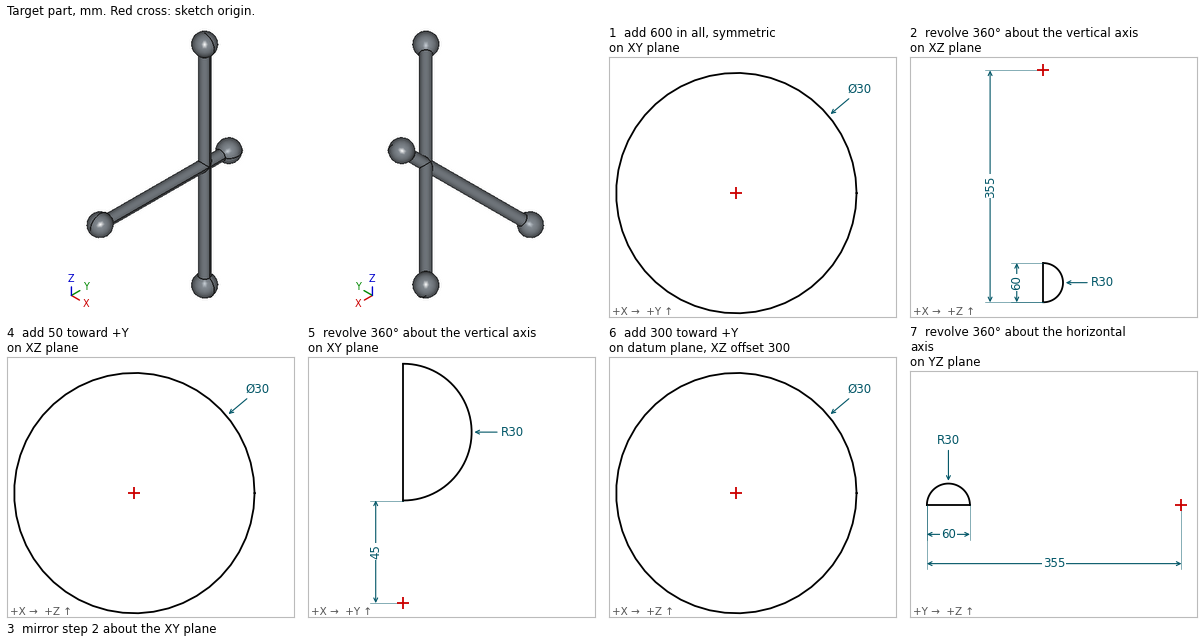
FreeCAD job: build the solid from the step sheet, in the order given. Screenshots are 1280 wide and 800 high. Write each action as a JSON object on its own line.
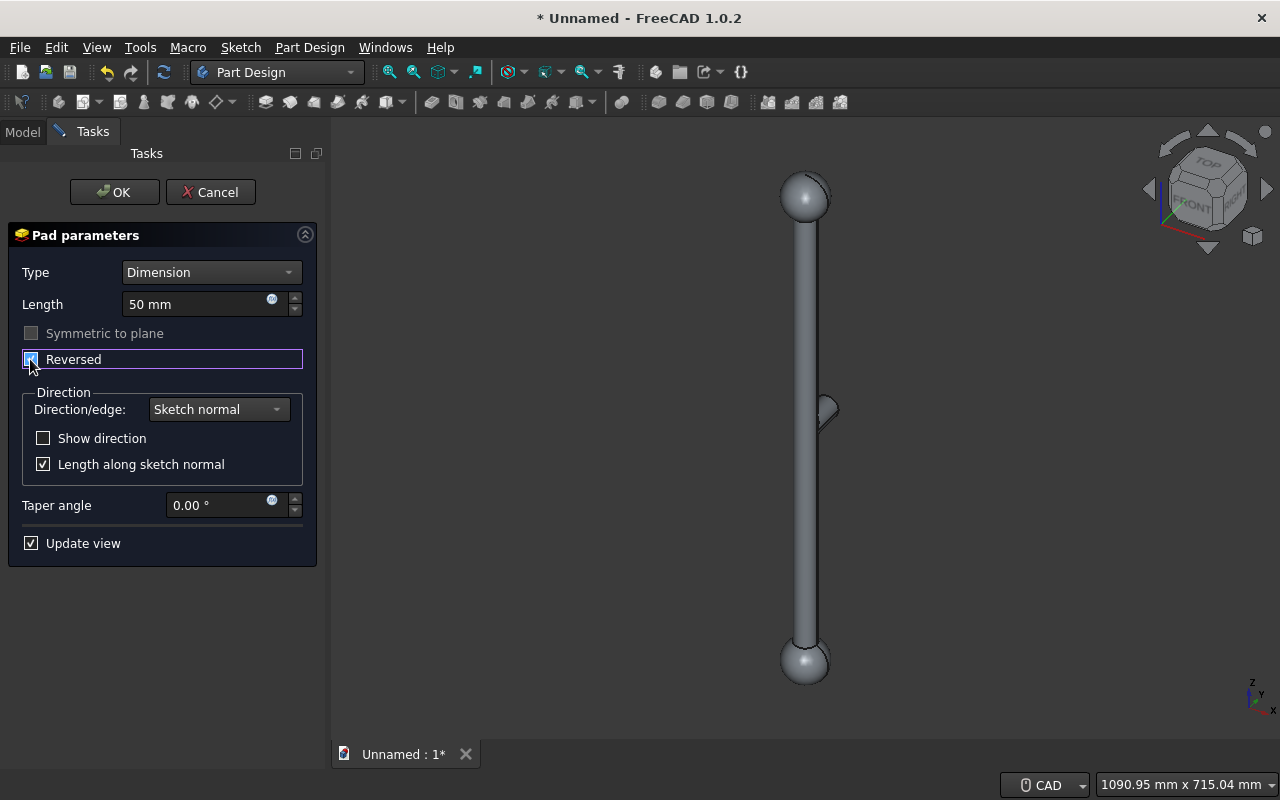
{"action": "left_click", "coordinate": [115, 192]}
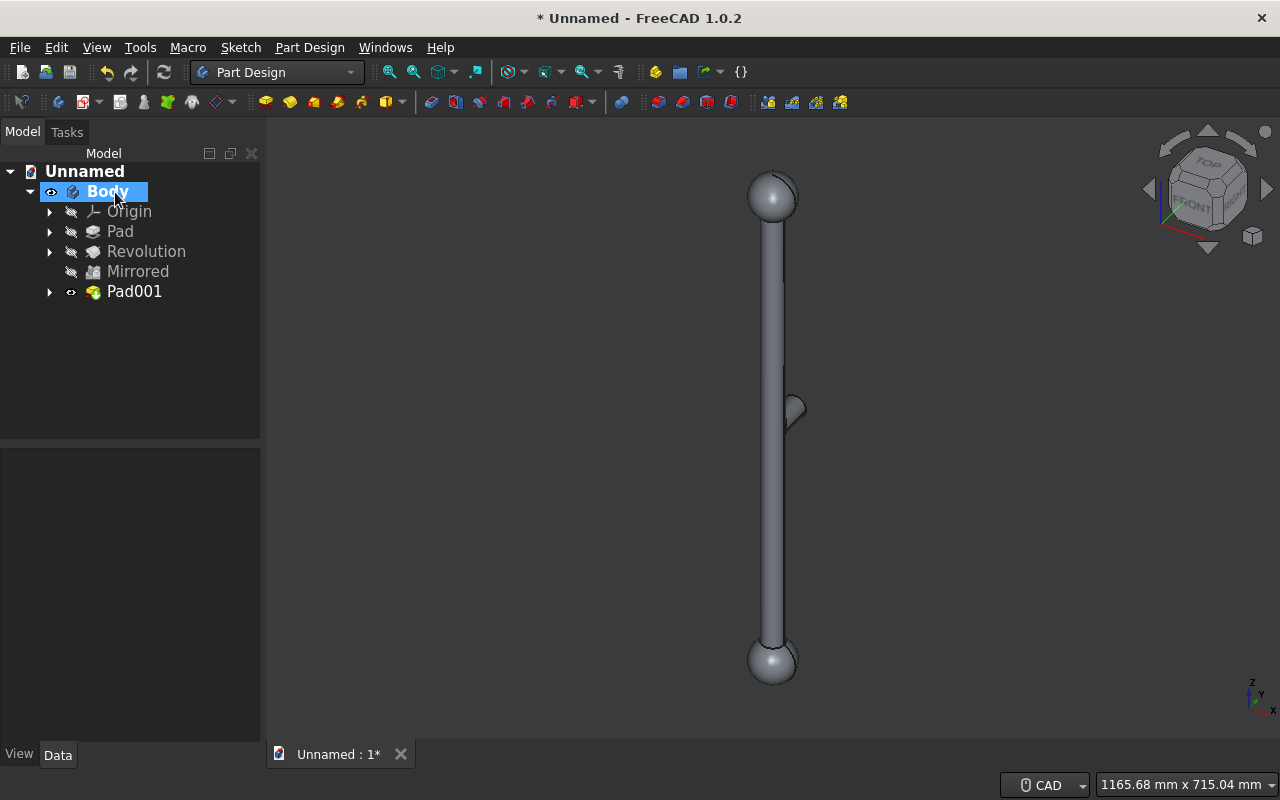
{"action": "left_click", "coordinate": [84, 102]}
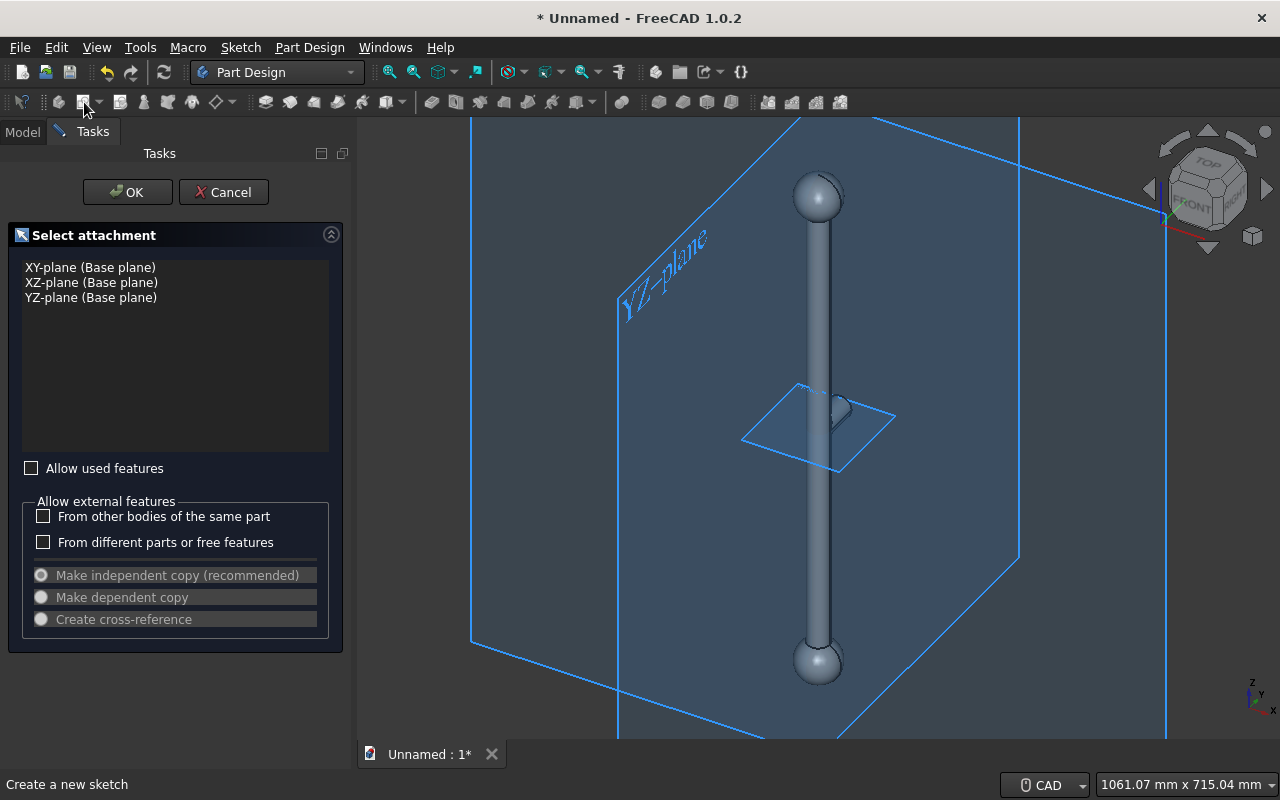
{"action": "left_click", "coordinate": [82, 268]}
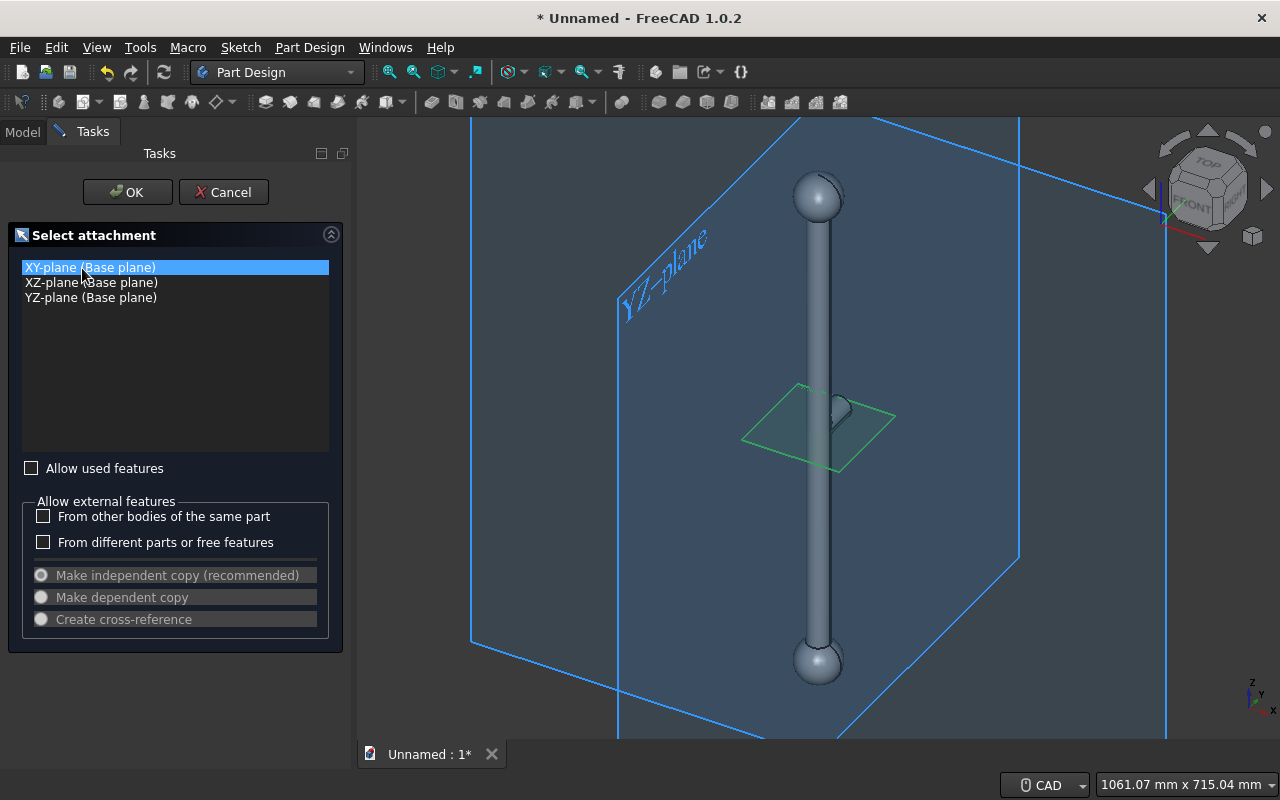
{"action": "left_click", "coordinate": [128, 192]}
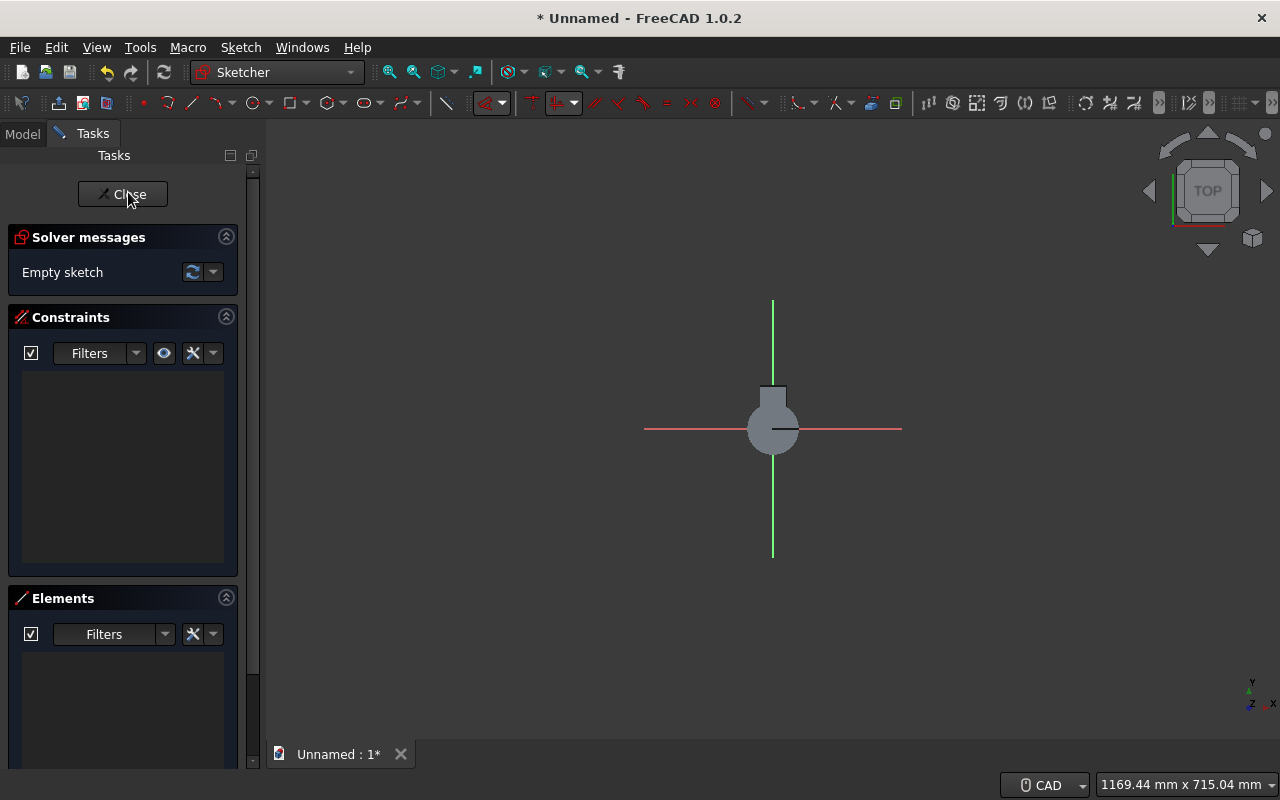
{"action": "left_click", "coordinate": [108, 104]}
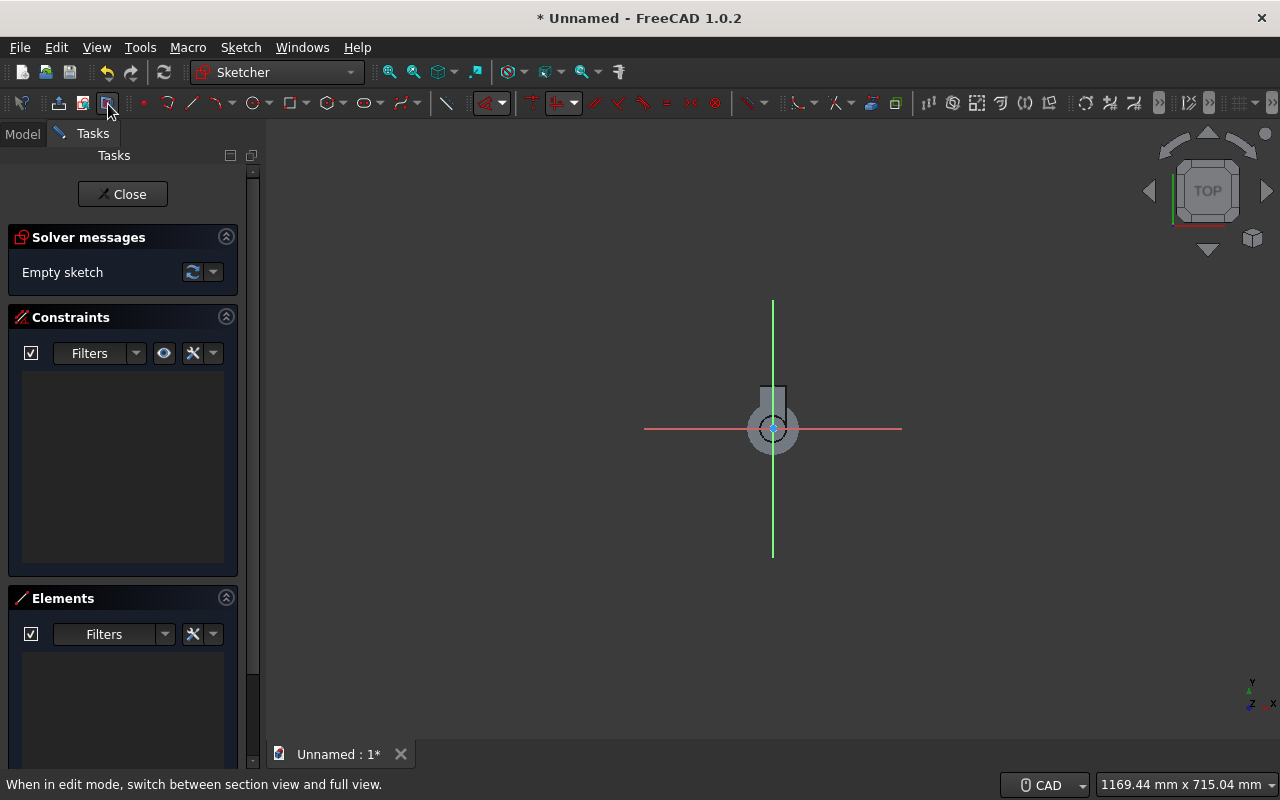
{"action": "scroll", "coordinate": [813, 369], "scroll_direction": "up", "scroll_amount": 7}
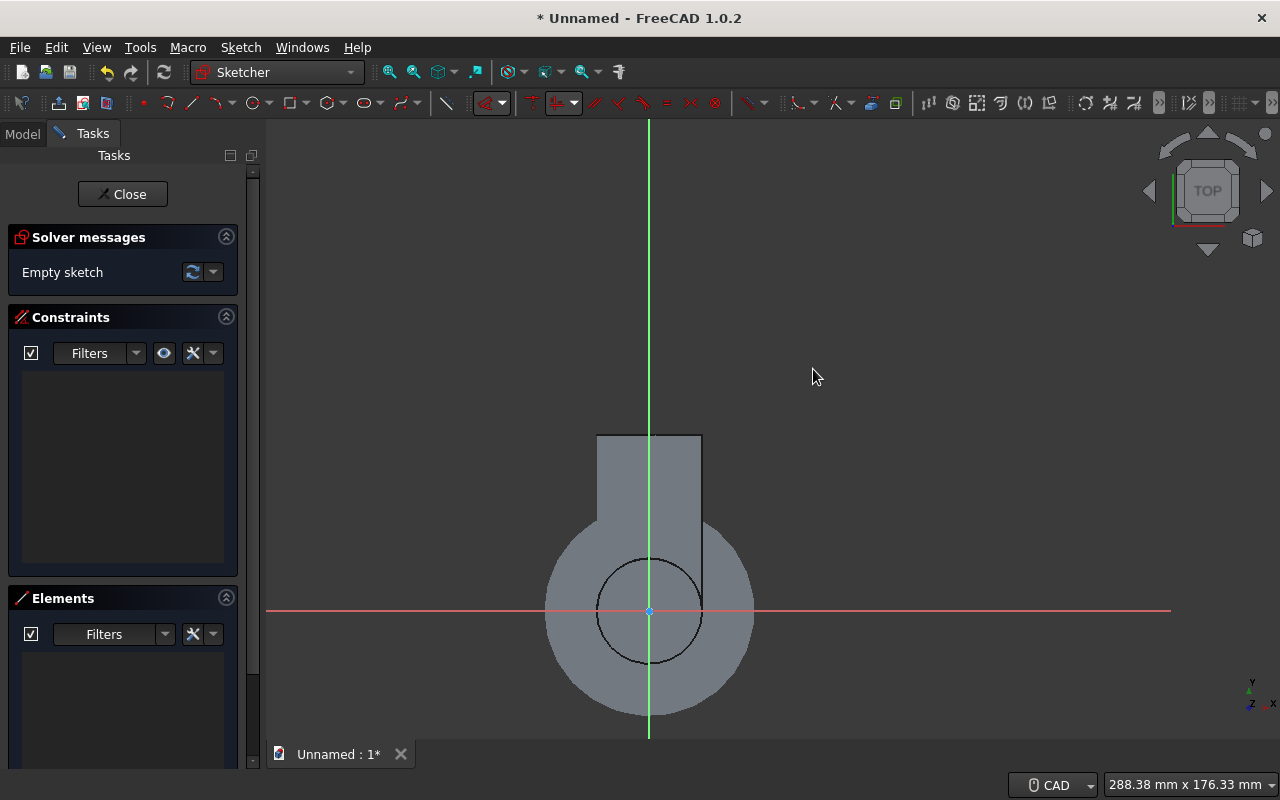
{"action": "left_click", "coordinate": [192, 104]}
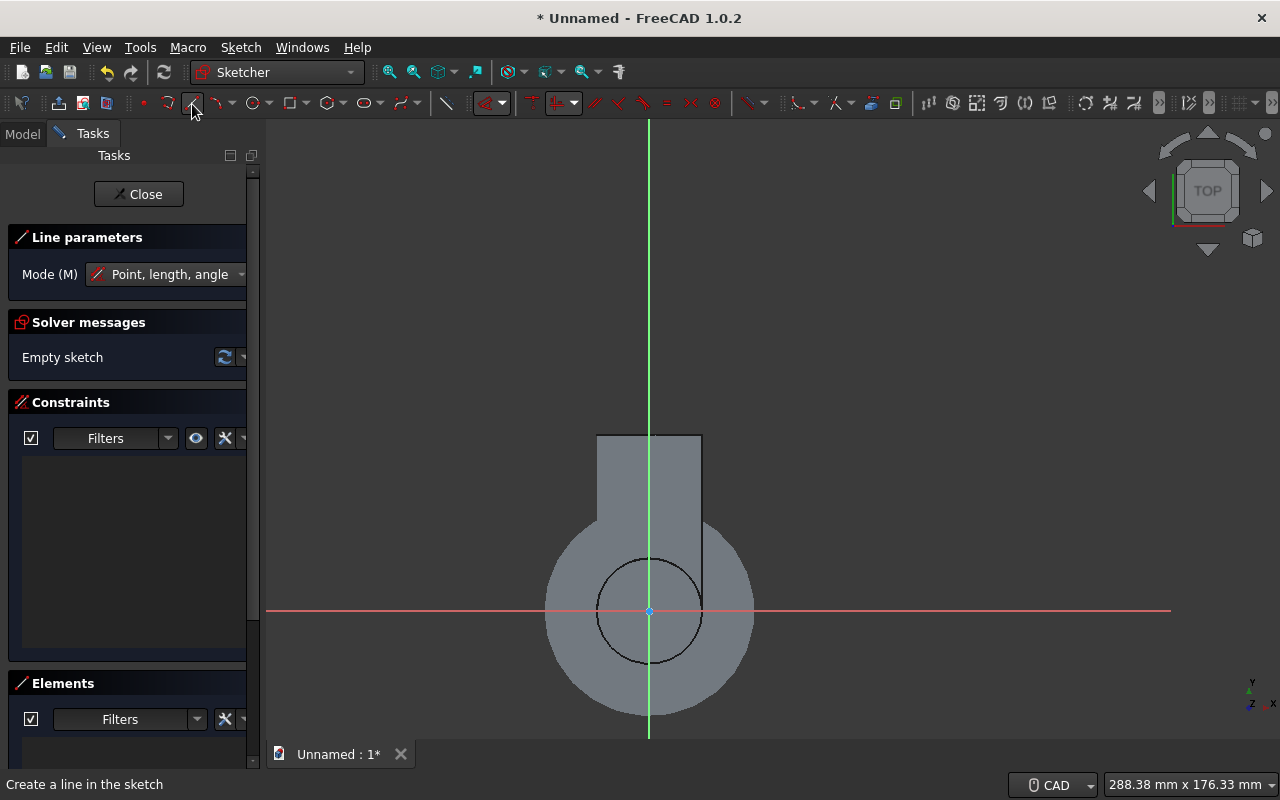
{"action": "left_click", "coordinate": [649, 242]}
{"action": "left_click", "coordinate": [658, 453]}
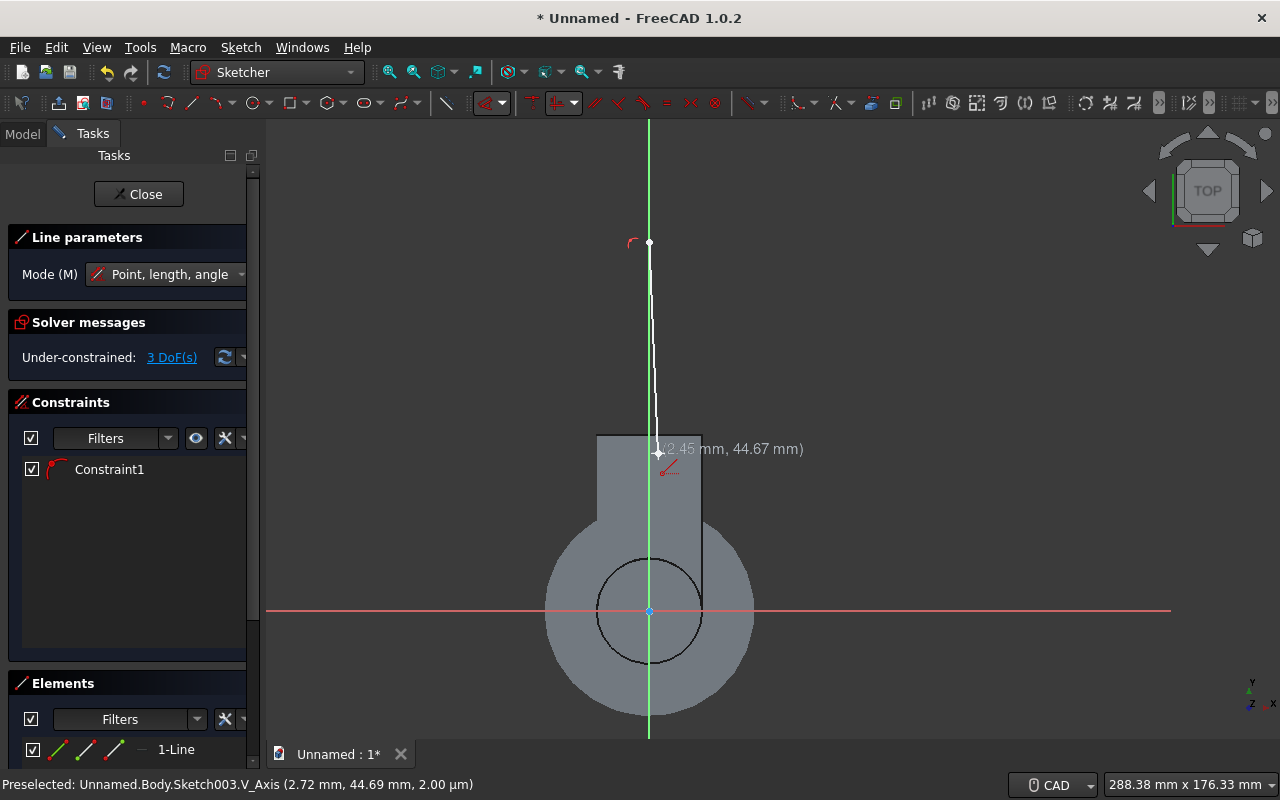
{"action": "key", "text": "g 3 a"}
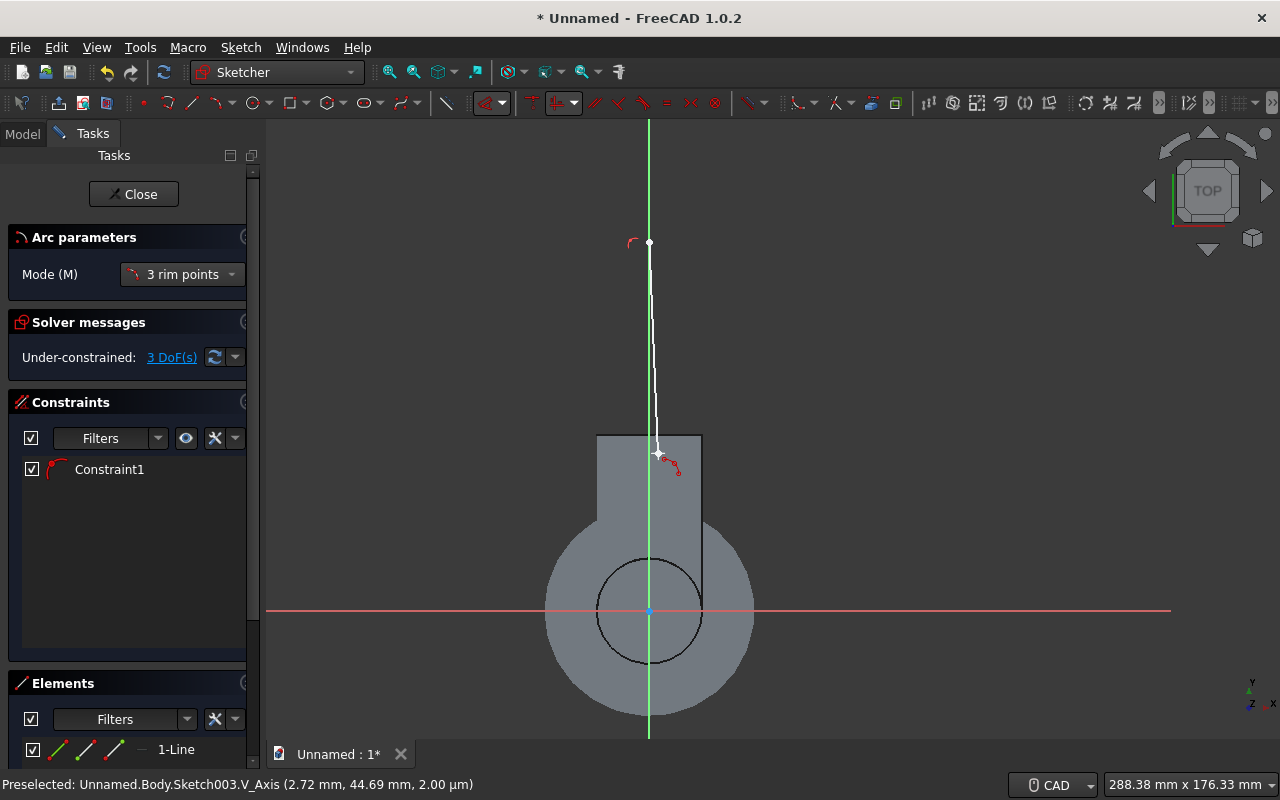
{"action": "left_click", "coordinate": [658, 454]}
{"action": "left_click", "coordinate": [649, 243]}
{"action": "left_click", "coordinate": [755, 347]}
{"action": "key", "text": "Escape"}